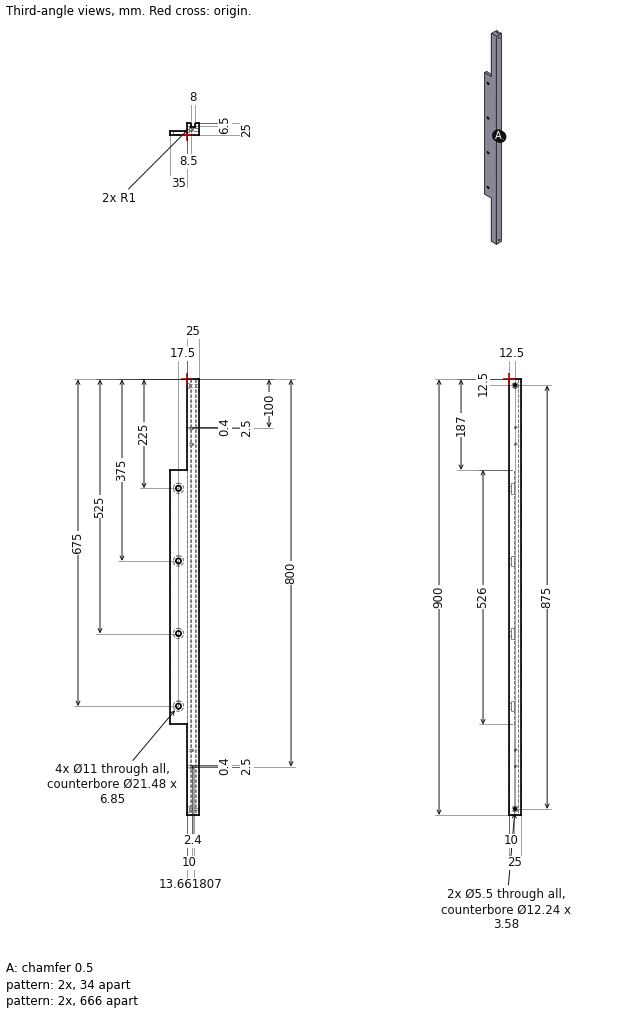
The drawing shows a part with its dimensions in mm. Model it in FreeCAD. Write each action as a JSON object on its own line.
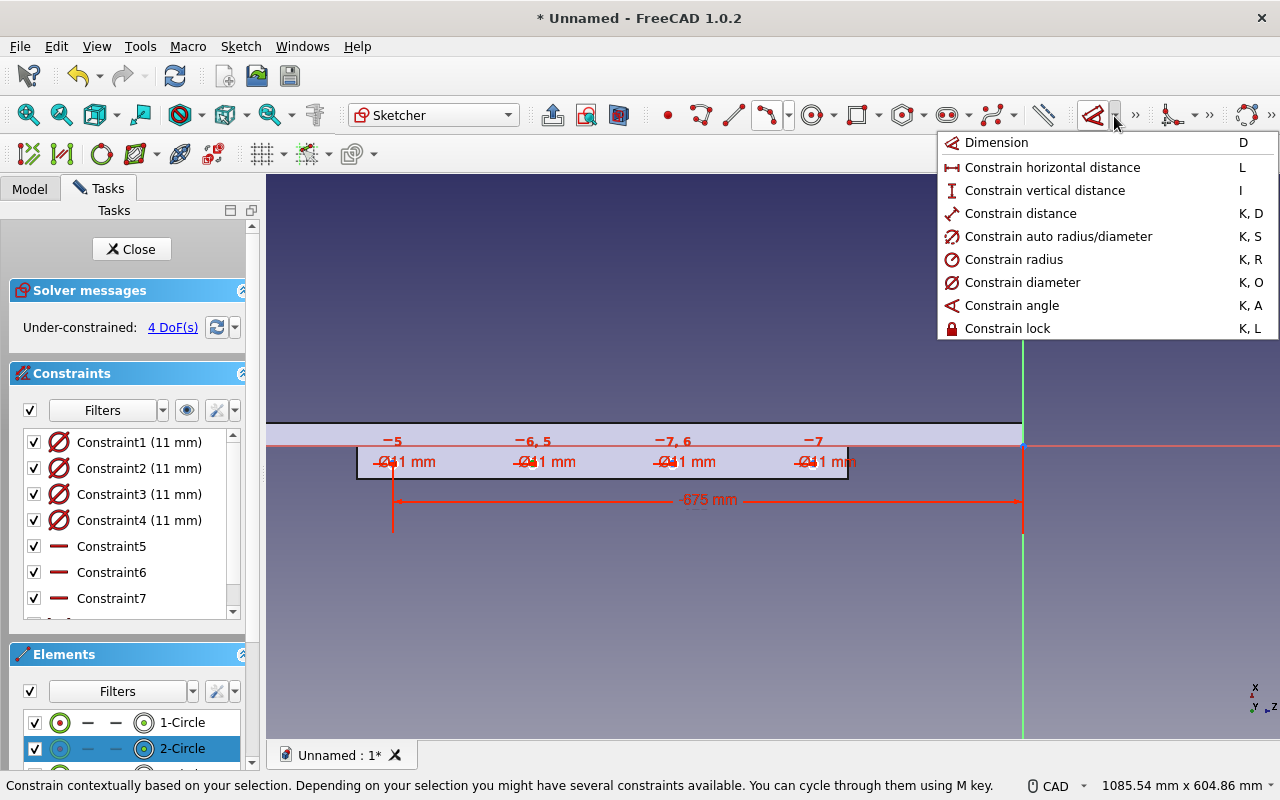
{"action": "left_click", "coordinate": [1108, 168]}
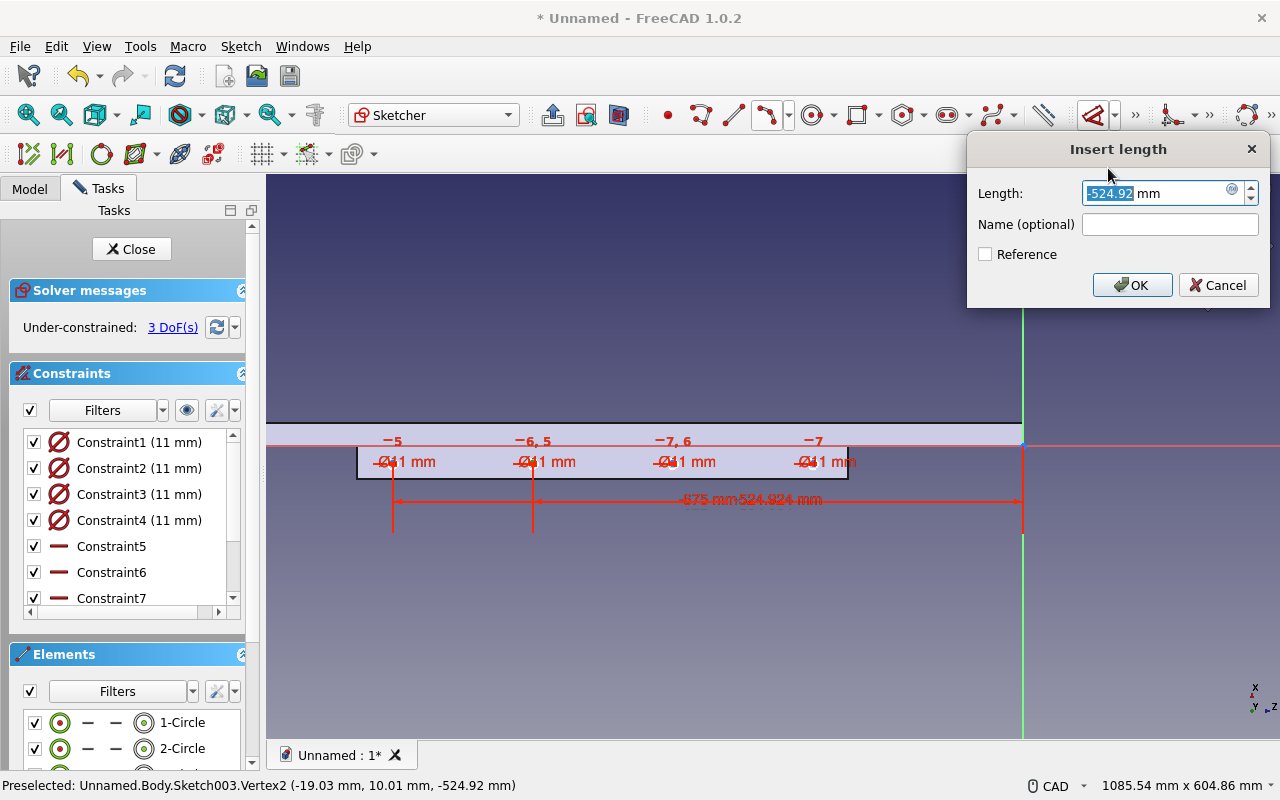
{"action": "type", "text": "-525"}
{"action": "key", "text": "Return"}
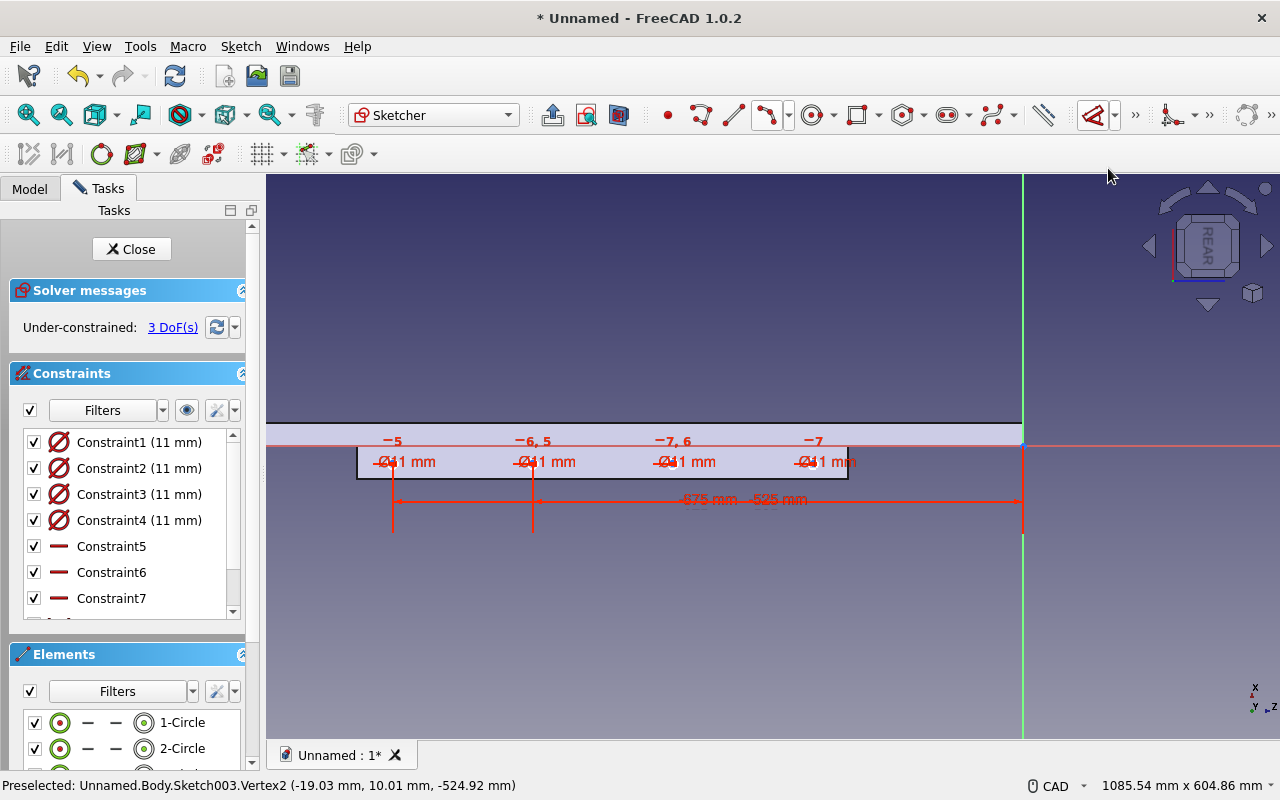
{"action": "left_click", "coordinate": [673, 464]}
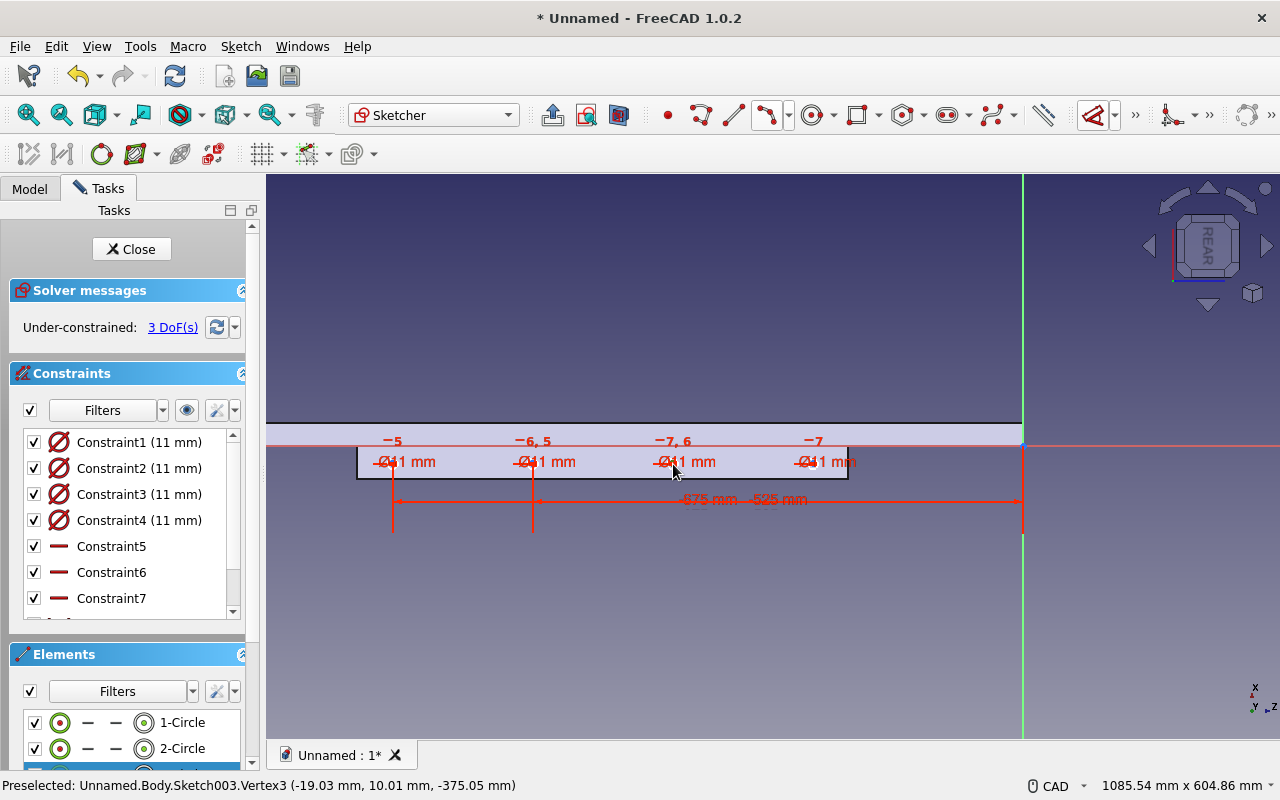
{"action": "left_click", "coordinate": [1114, 116]}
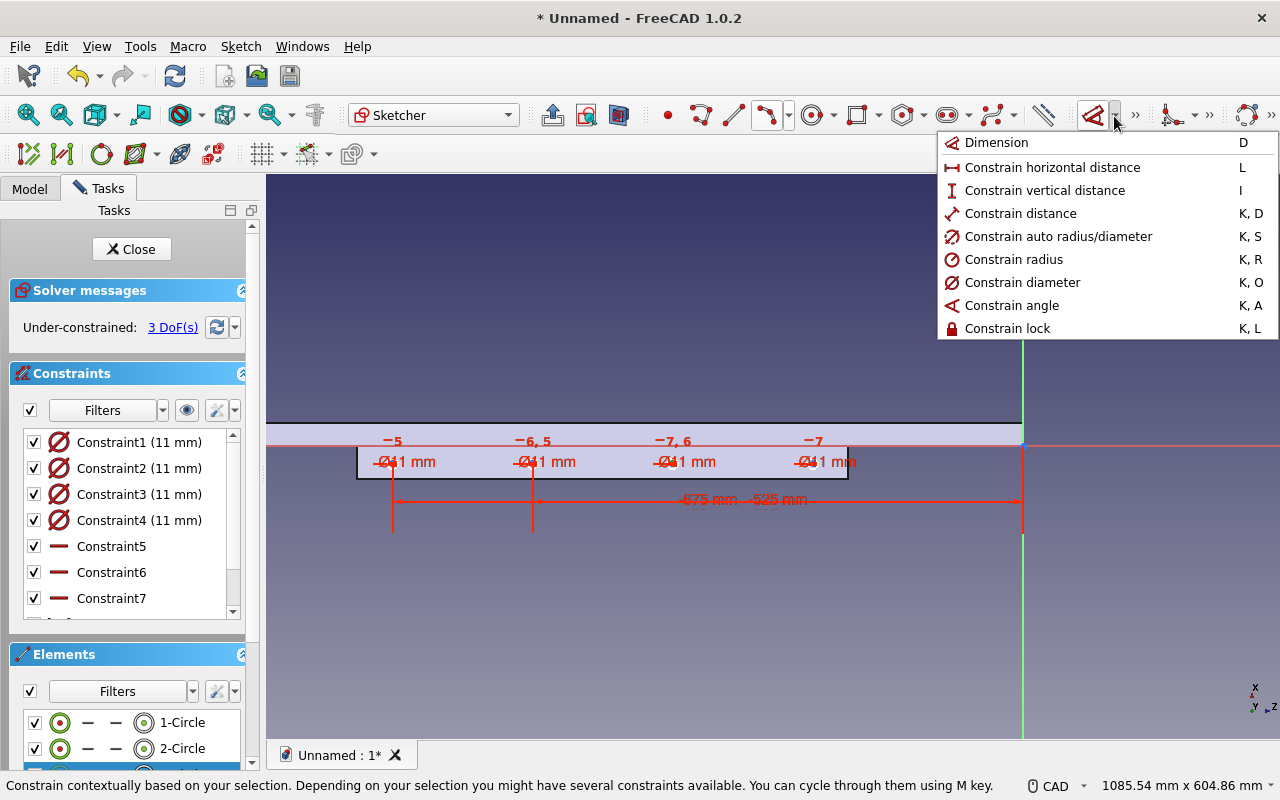
{"action": "left_click", "coordinate": [1108, 168]}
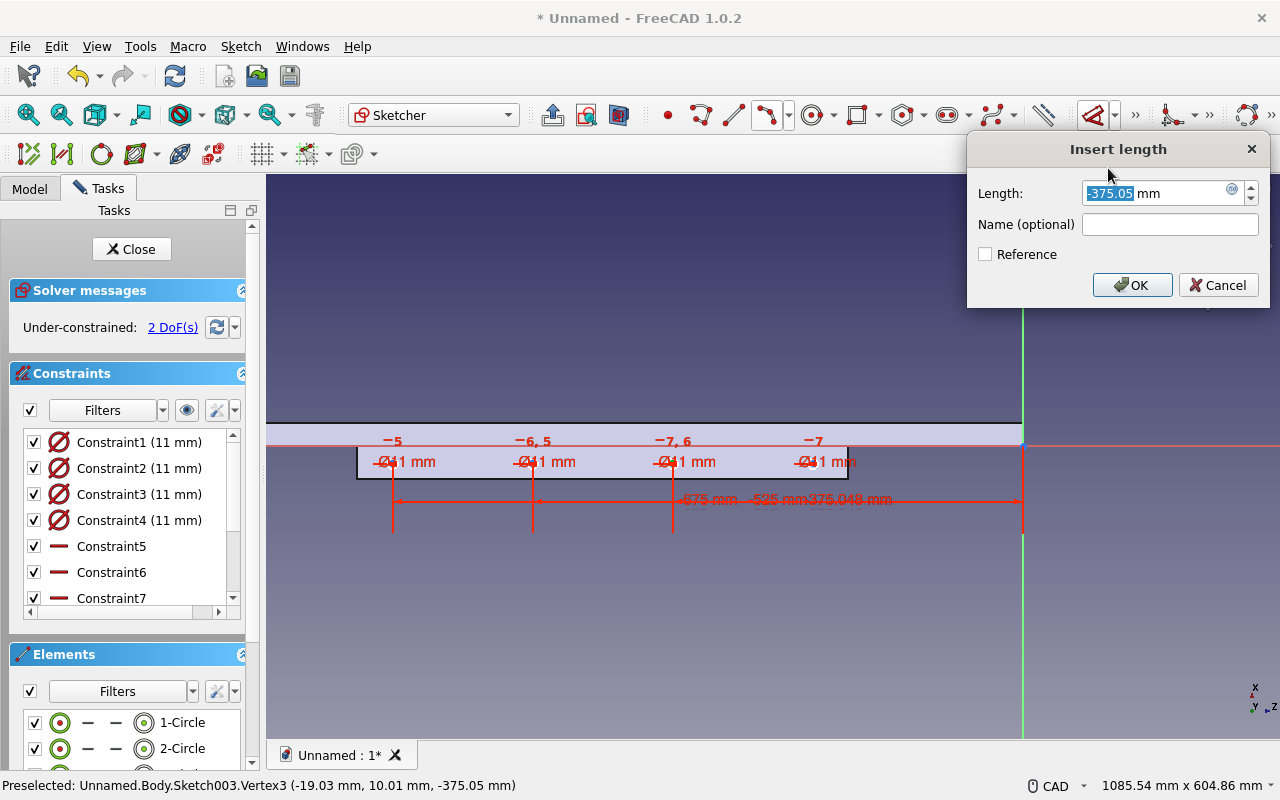
{"action": "type", "text": "-375"}
{"action": "key", "text": "Return"}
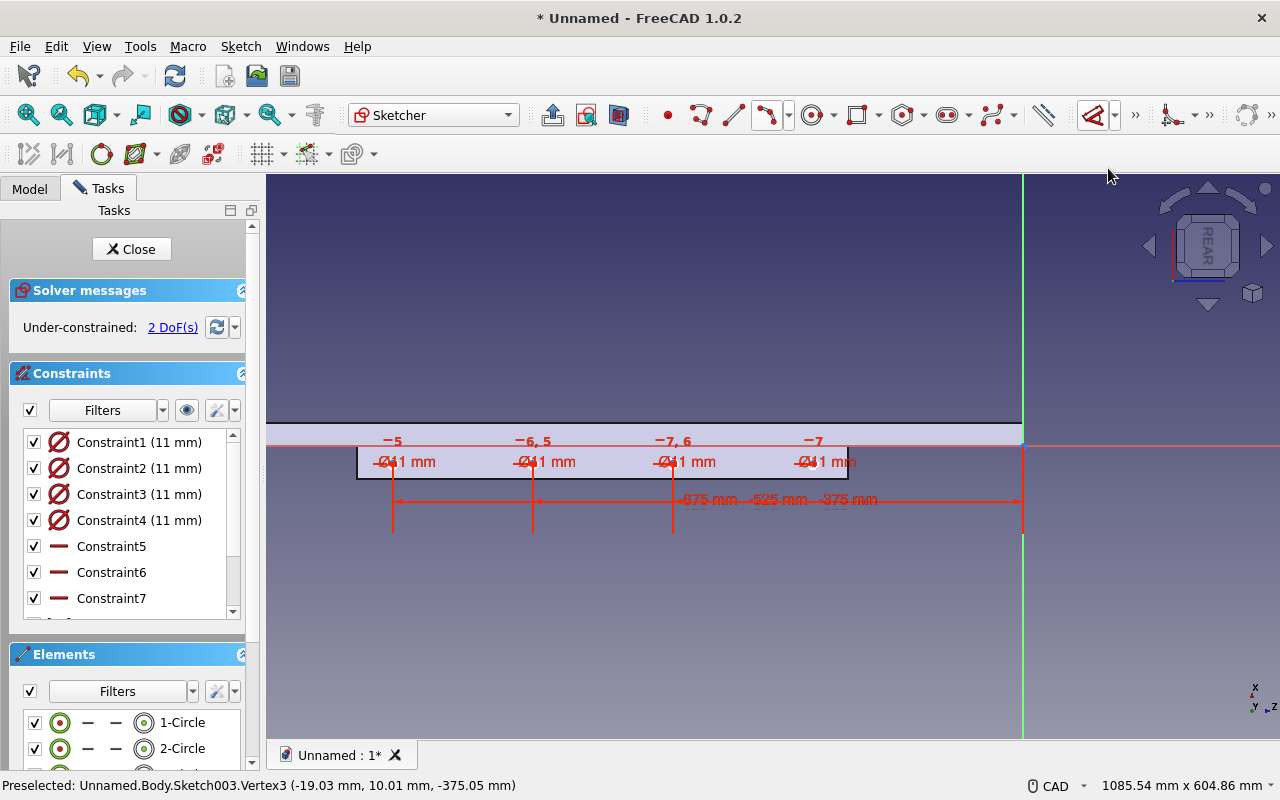
{"action": "left_click", "coordinate": [813, 464]}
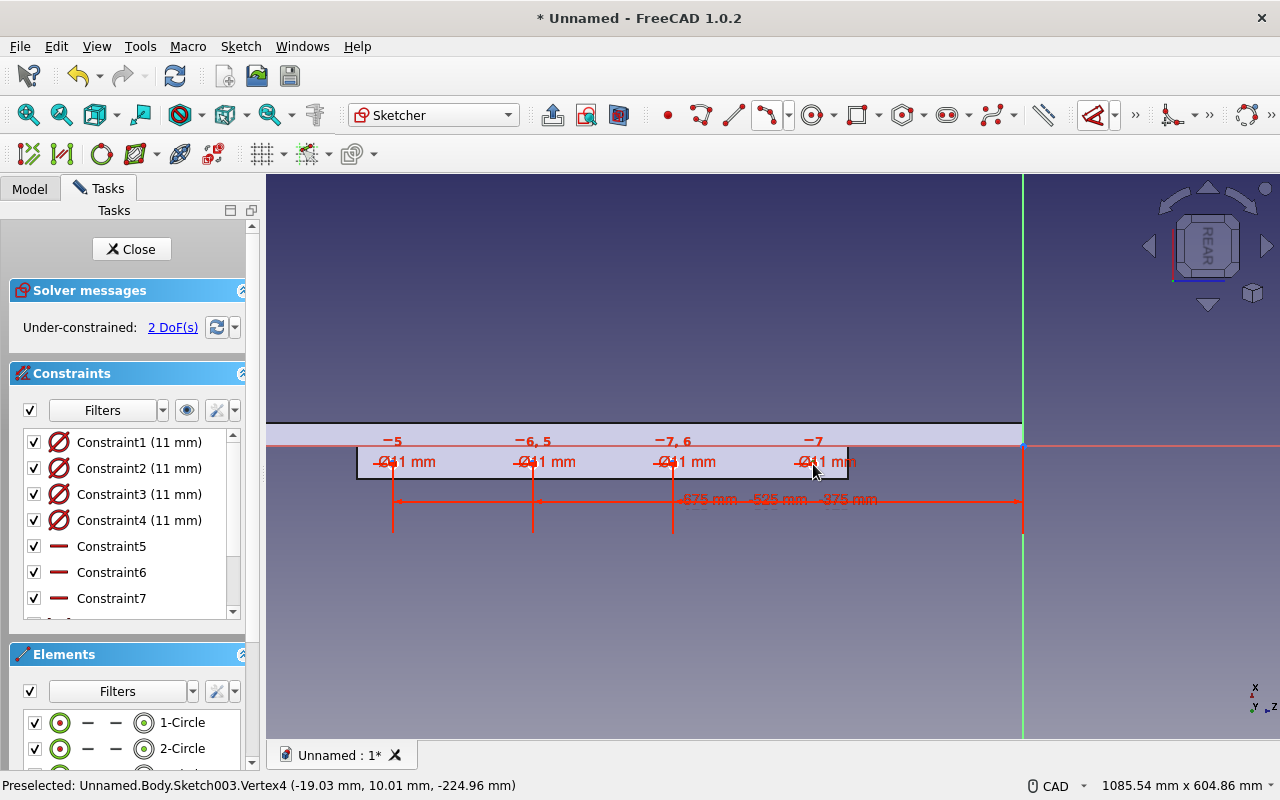
{"action": "left_click", "coordinate": [1114, 116]}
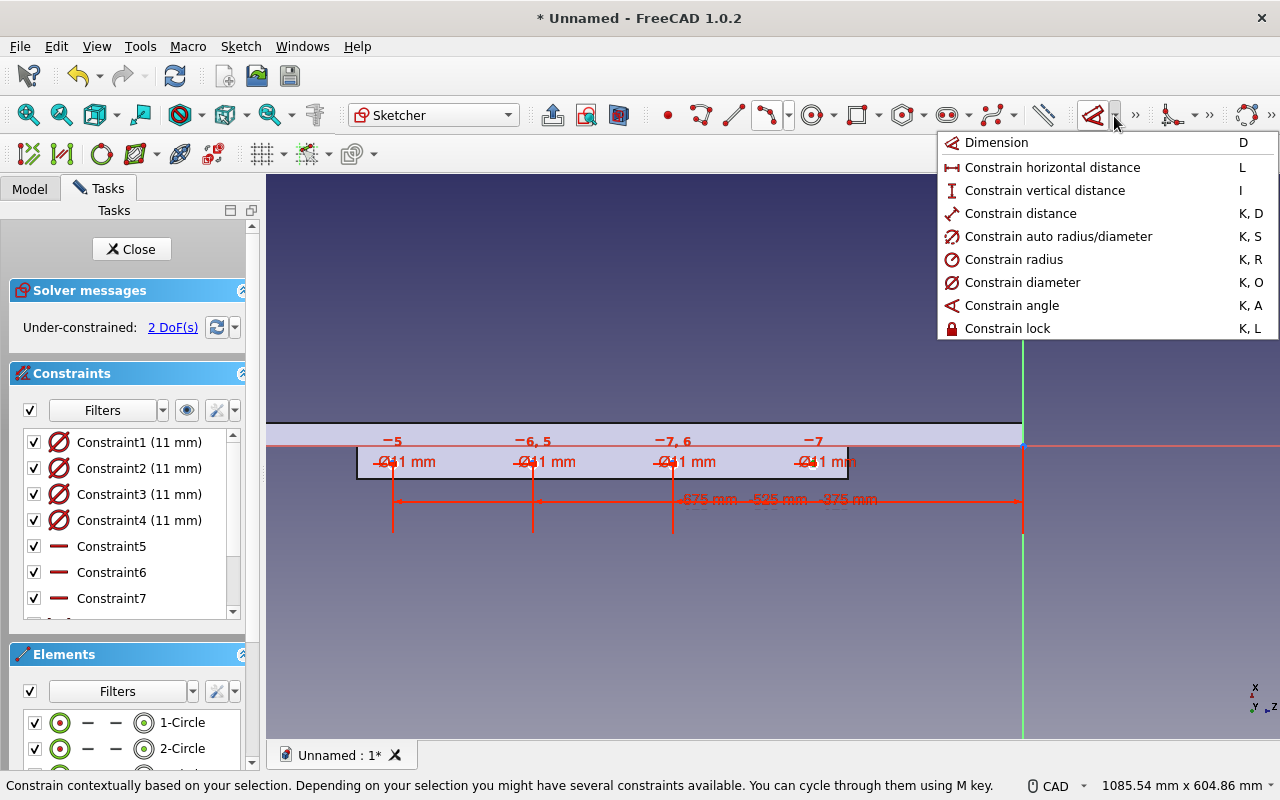
{"action": "left_click", "coordinate": [1108, 168]}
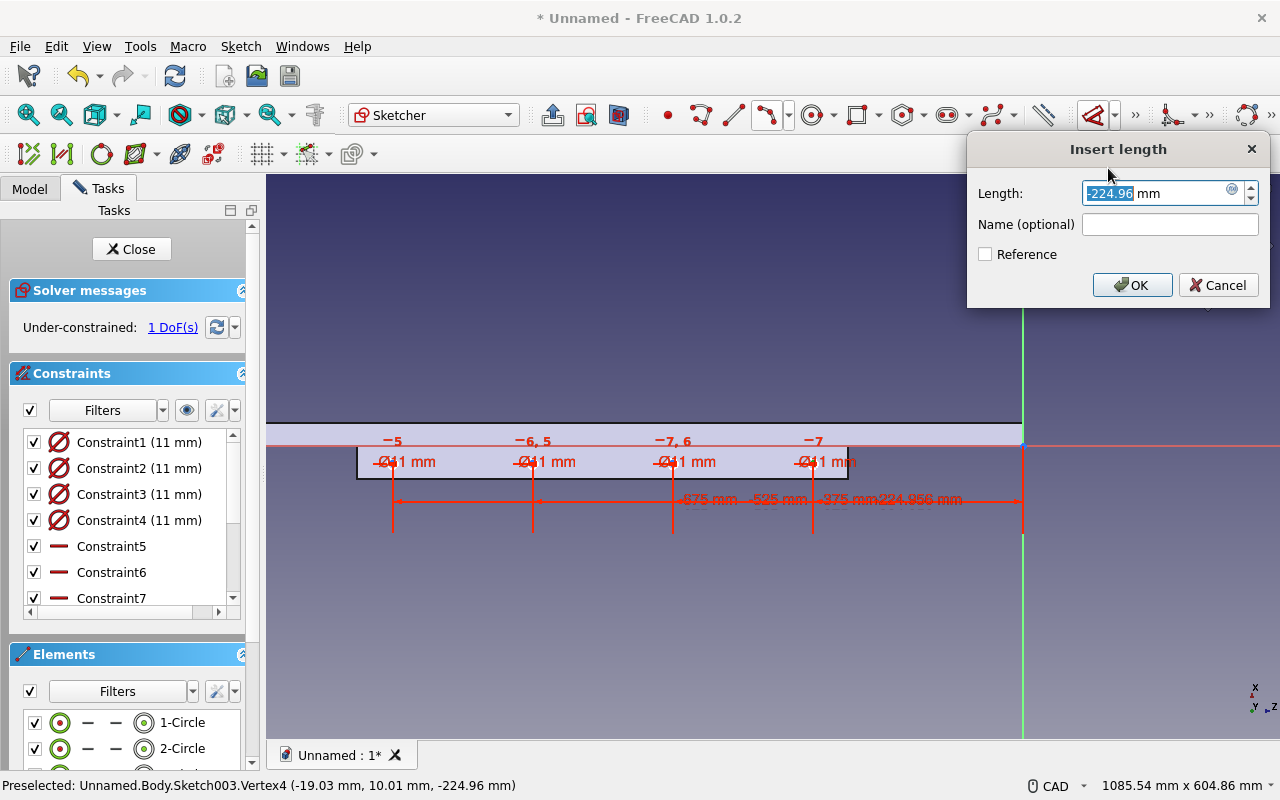
{"action": "type", "text": "-225"}
{"action": "key", "text": "Return"}